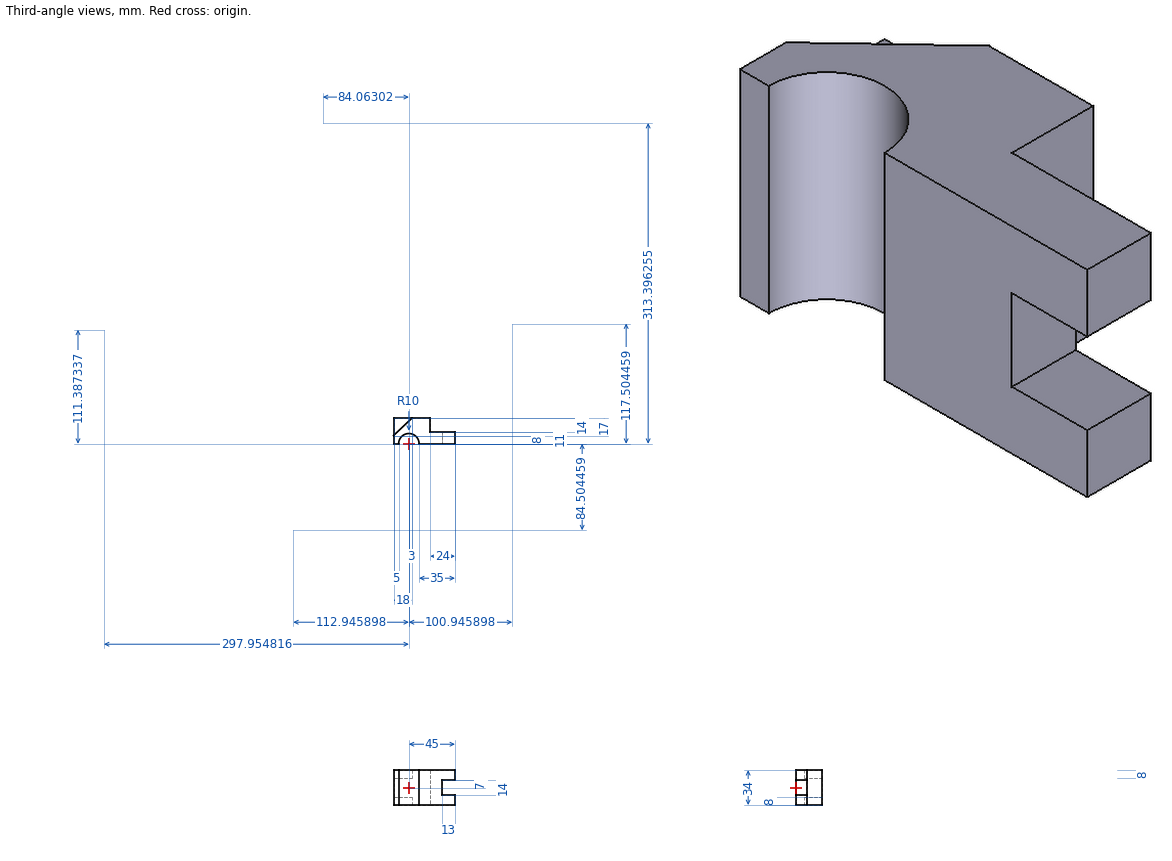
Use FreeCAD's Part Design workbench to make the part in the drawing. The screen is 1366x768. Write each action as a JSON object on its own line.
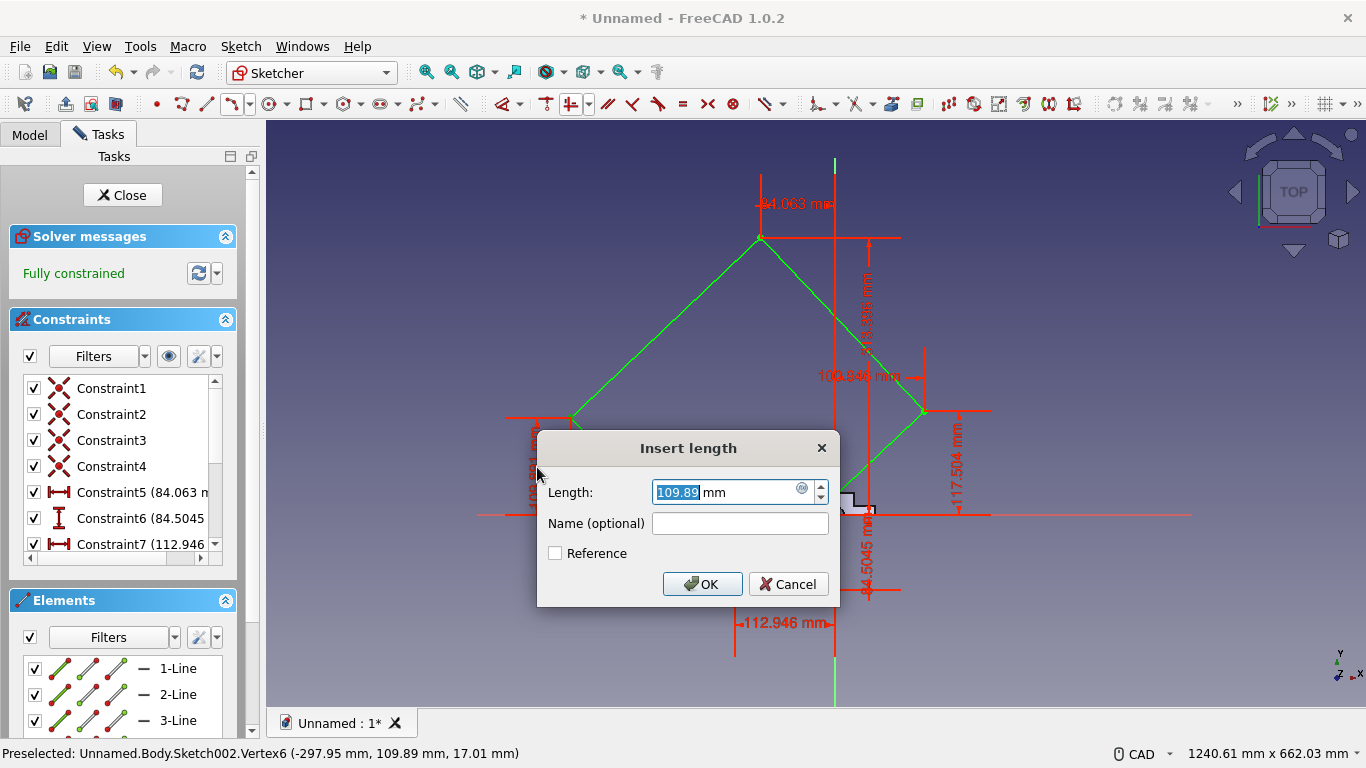
{"action": "type", "text": "111.387337"}
{"action": "key", "text": "Return"}
{"action": "key", "text": "Escape"}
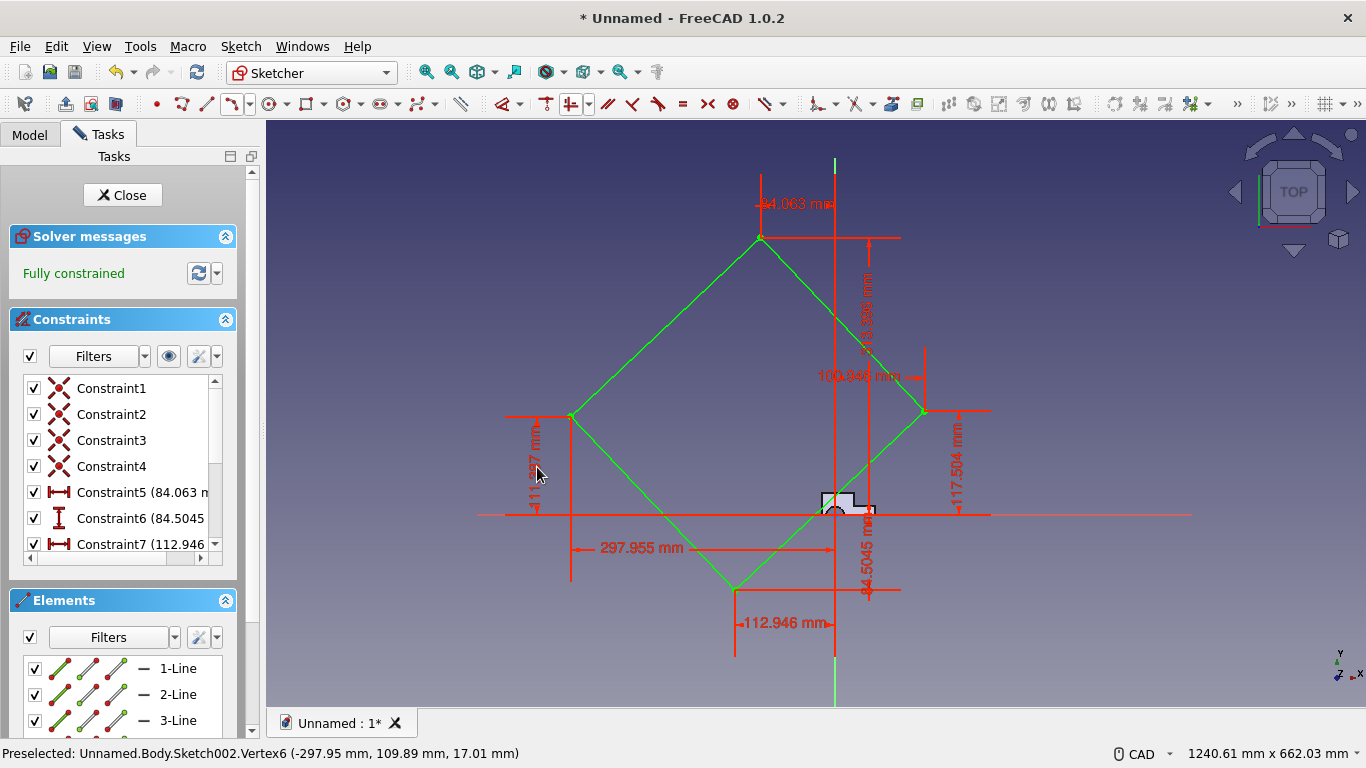
{"action": "left_click", "coordinate": [123, 195]}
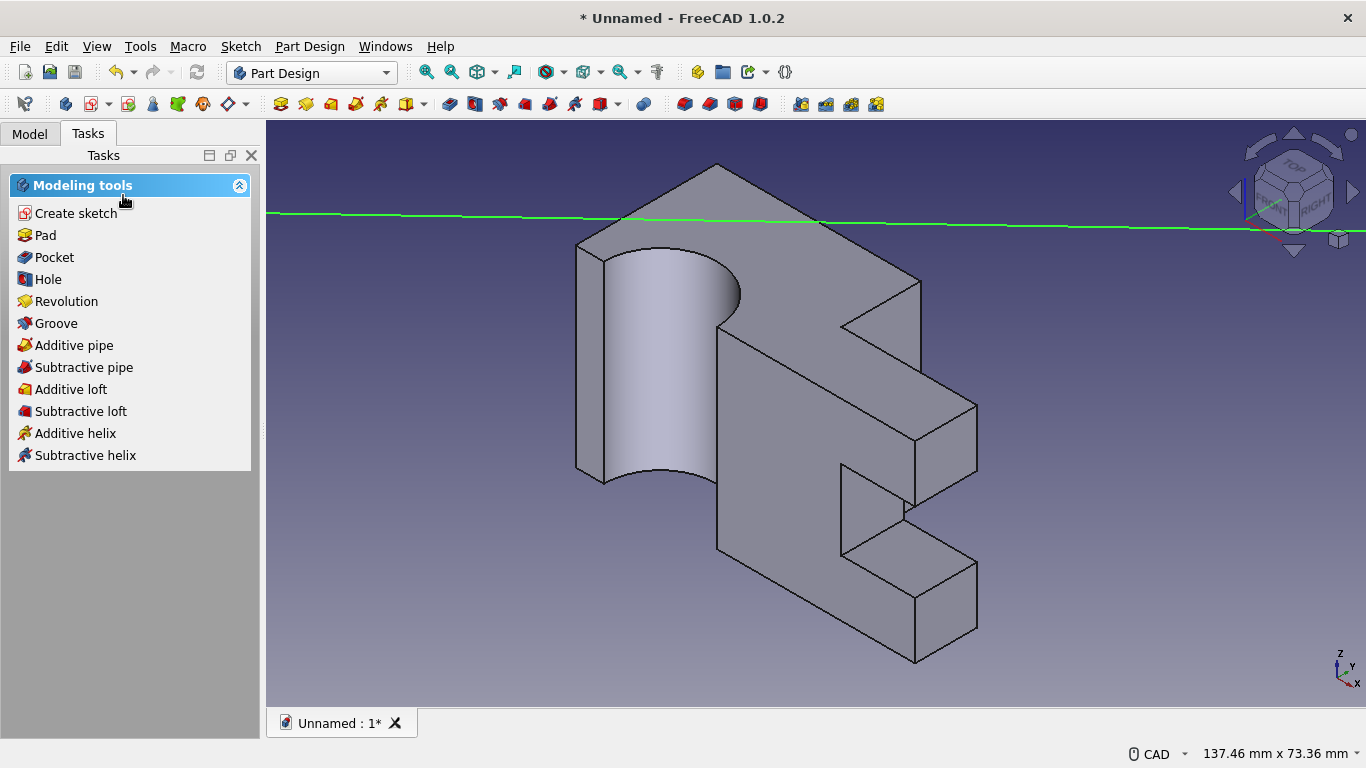
{"action": "left_click", "coordinate": [450, 104]}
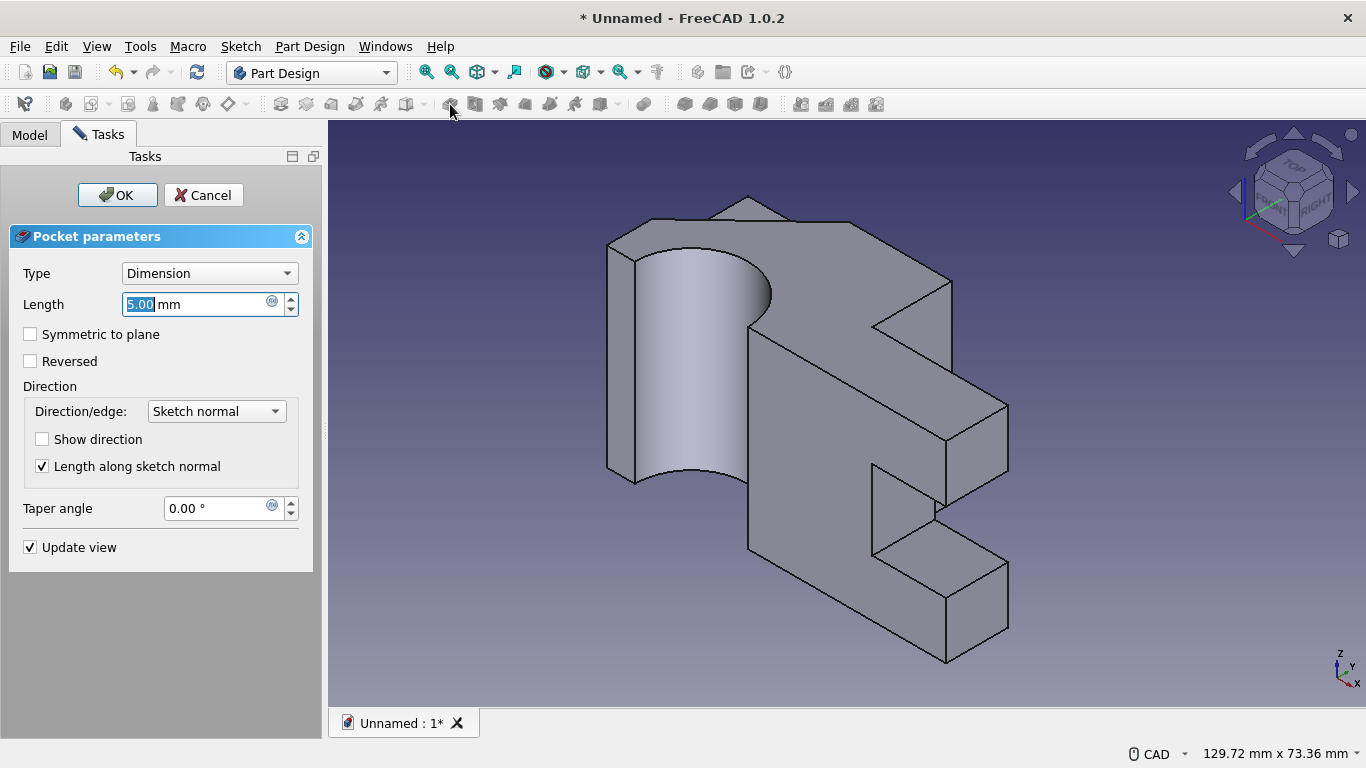
{"action": "left_click", "coordinate": [210, 274]}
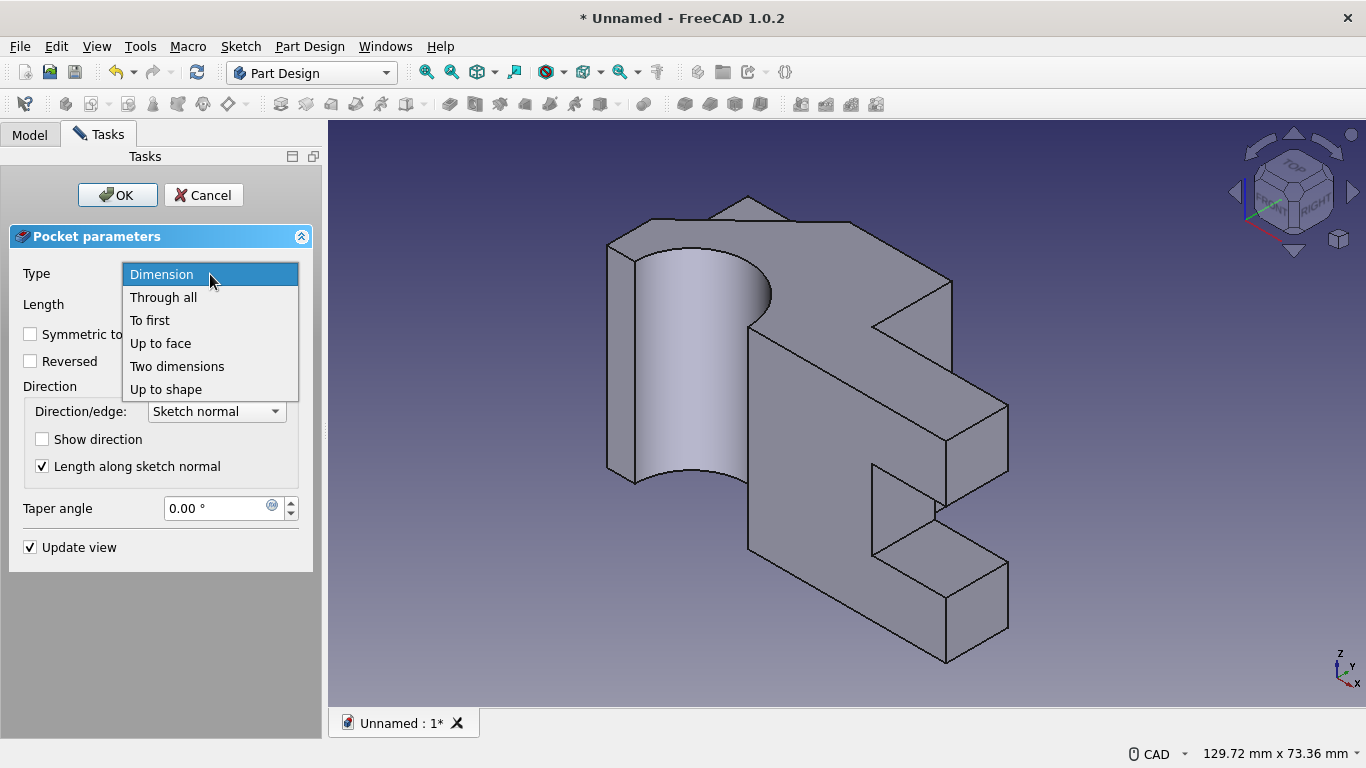
{"action": "left_click", "coordinate": [208, 366]}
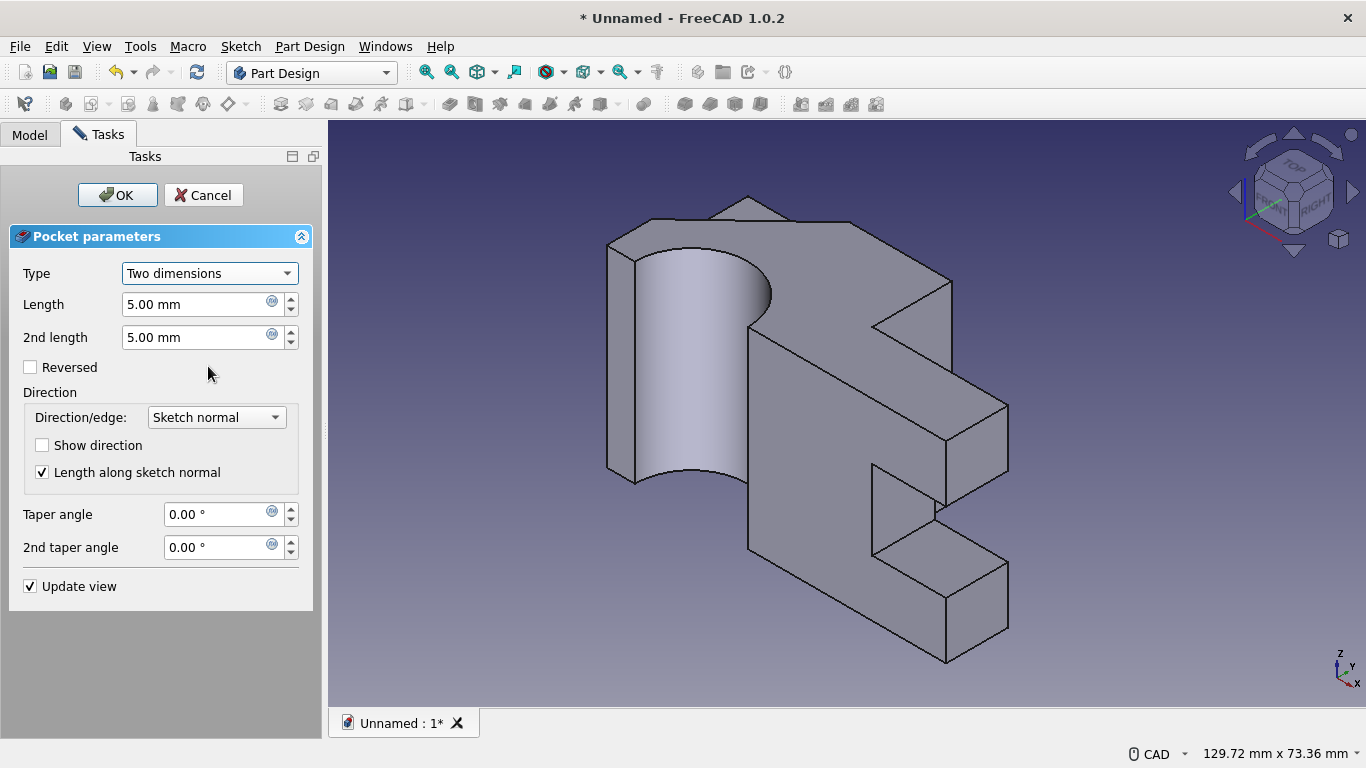
{"action": "triple_click", "coordinate": [204, 304]}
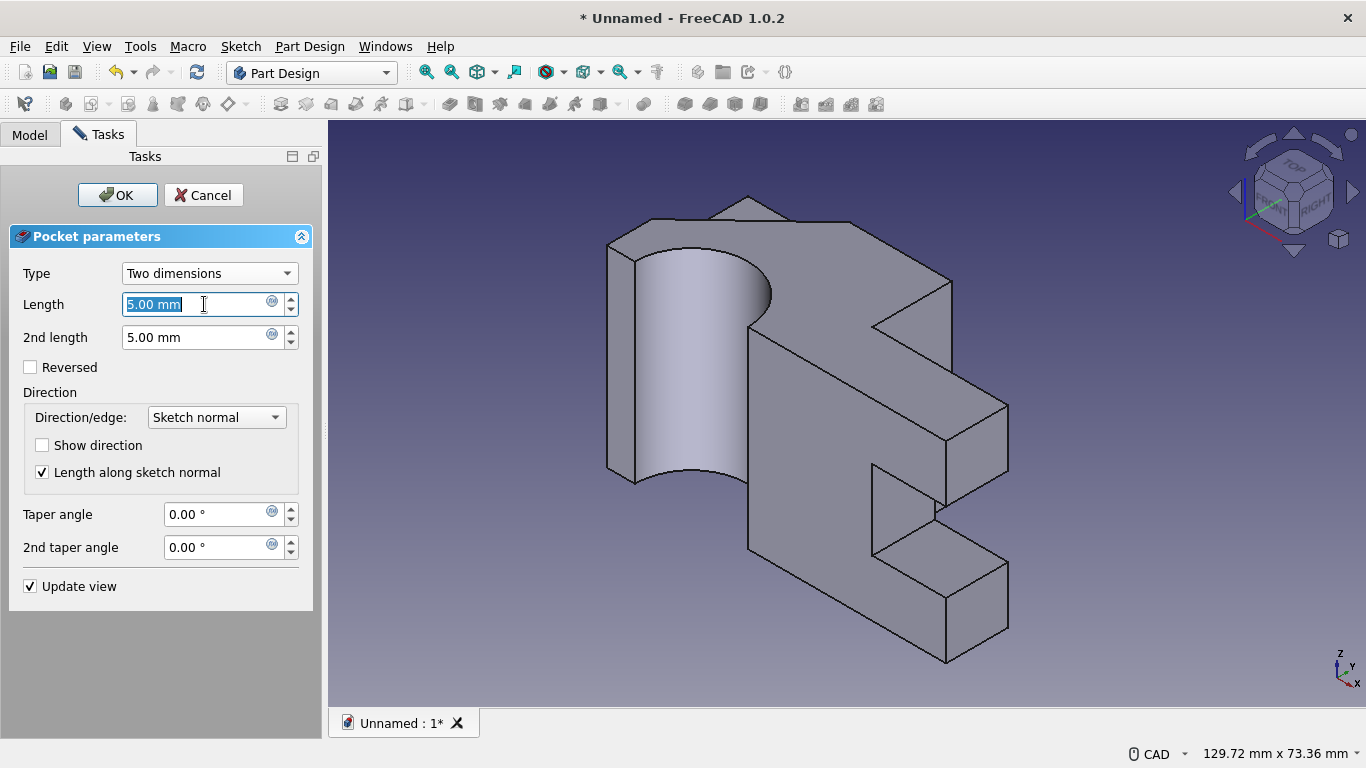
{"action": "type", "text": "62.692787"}
{"action": "key", "text": "Tab"}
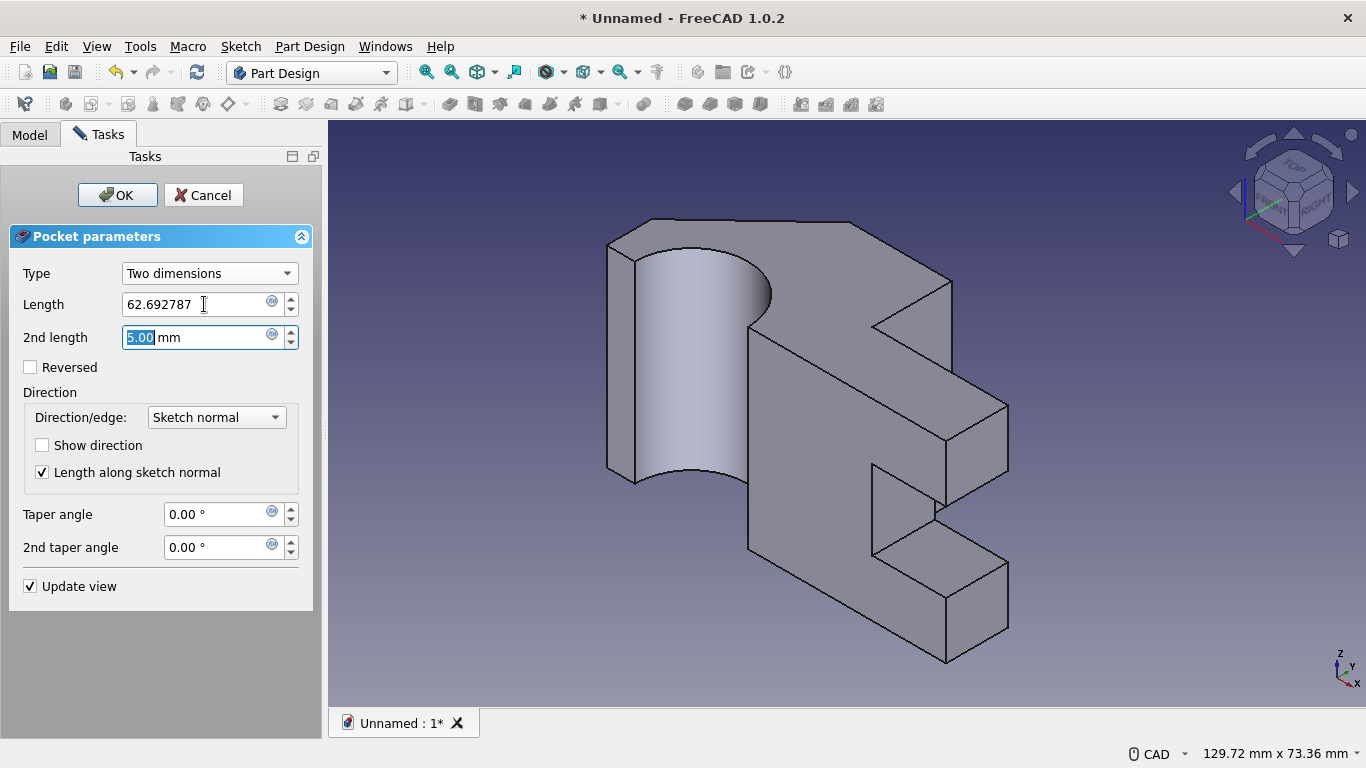
{"action": "type", "text": "8"}
{"action": "key", "text": "Tab"}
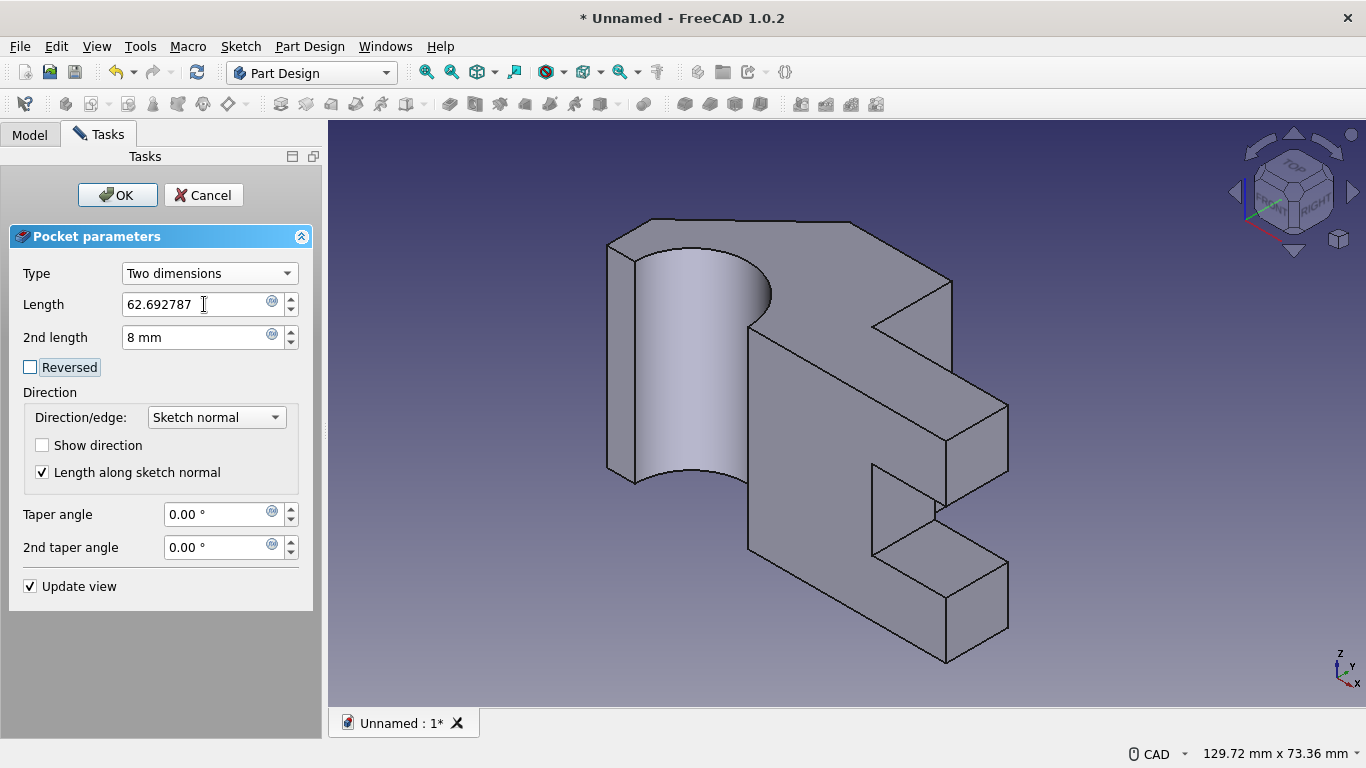
{"action": "left_click", "coordinate": [31, 367]}